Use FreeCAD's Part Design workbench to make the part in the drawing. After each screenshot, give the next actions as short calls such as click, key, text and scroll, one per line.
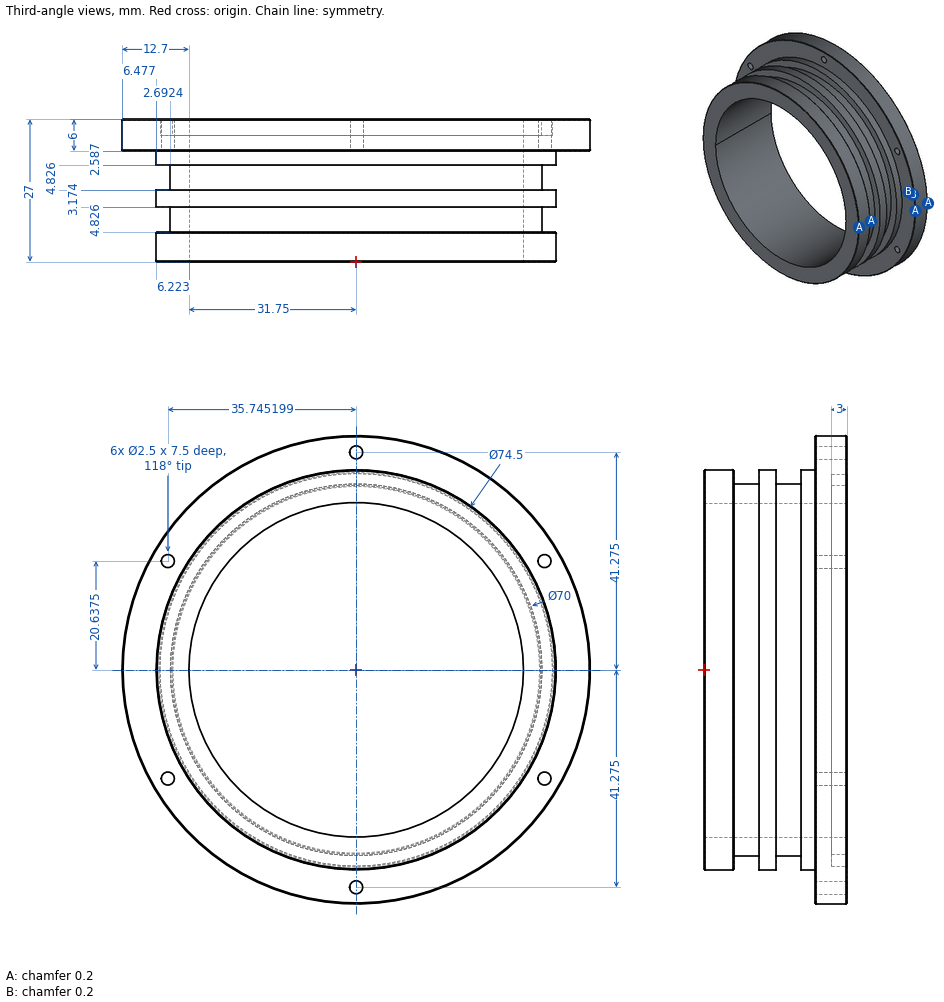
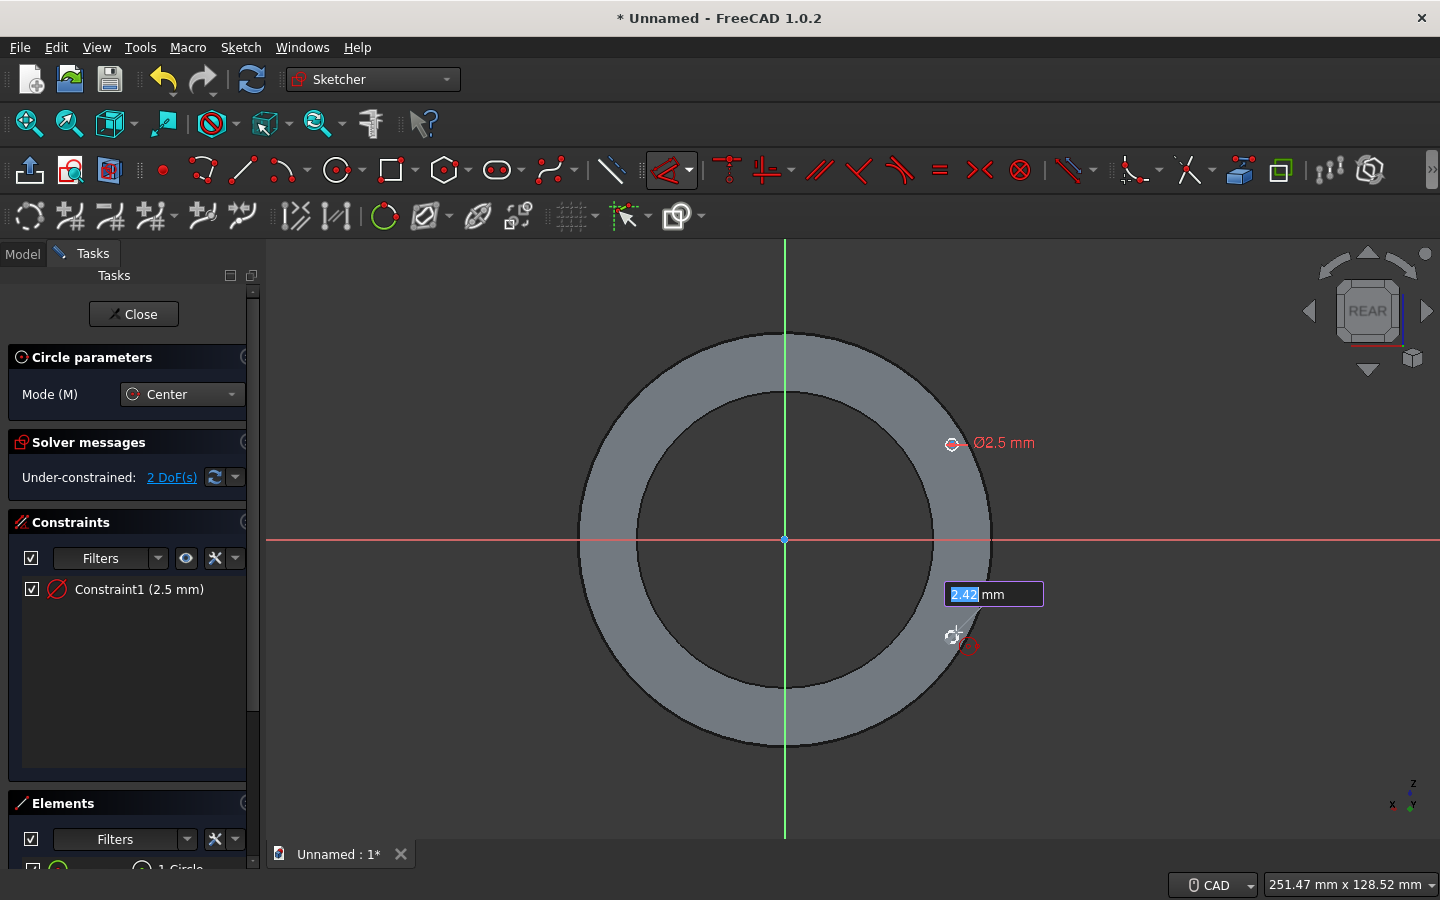
text(2.5)
key(Return)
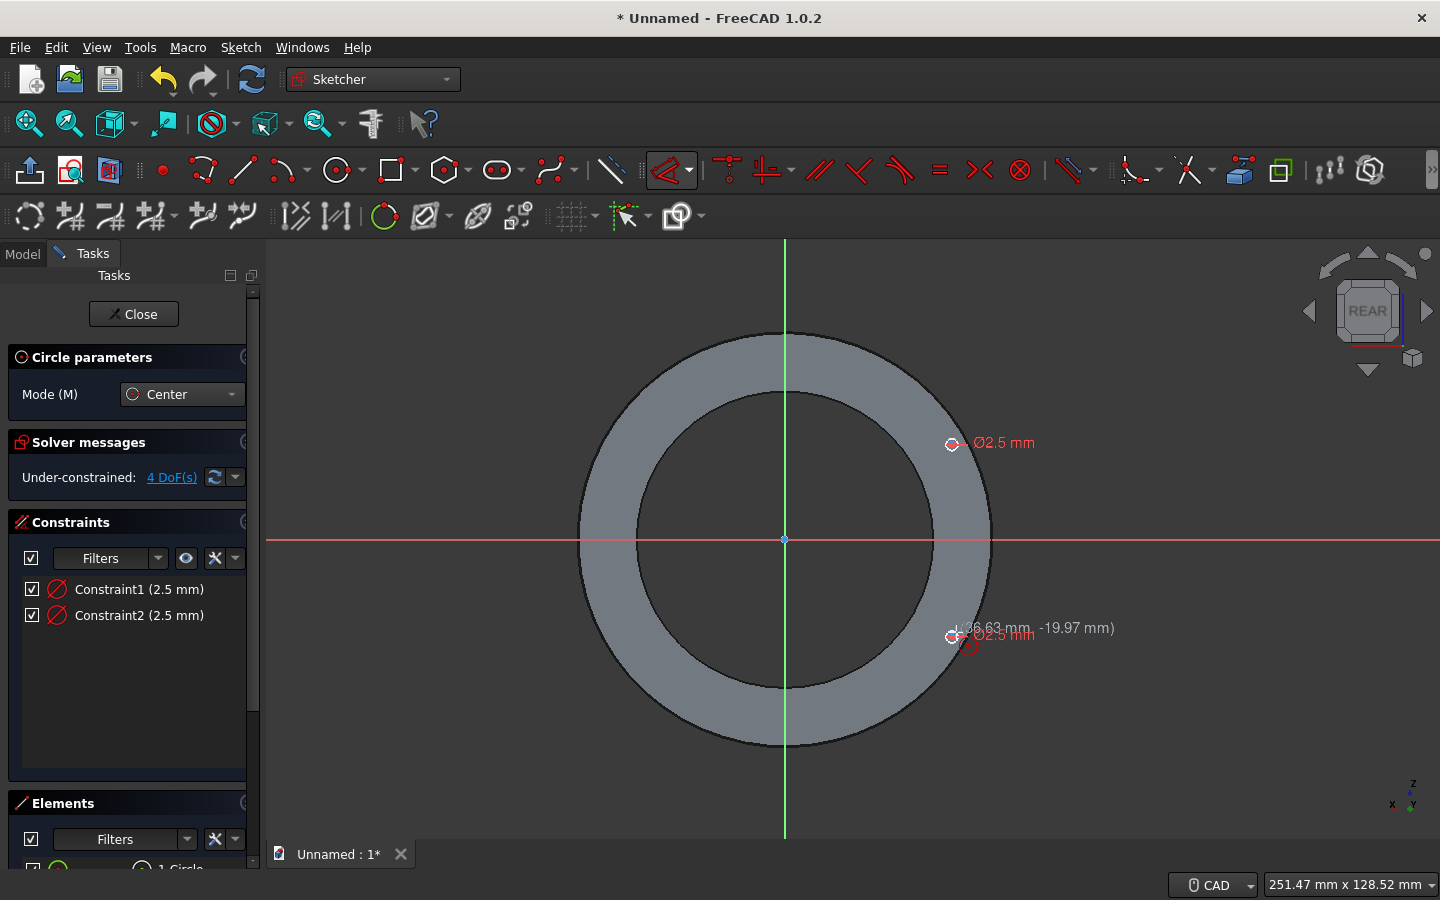
scroll(785, 732, up, 7)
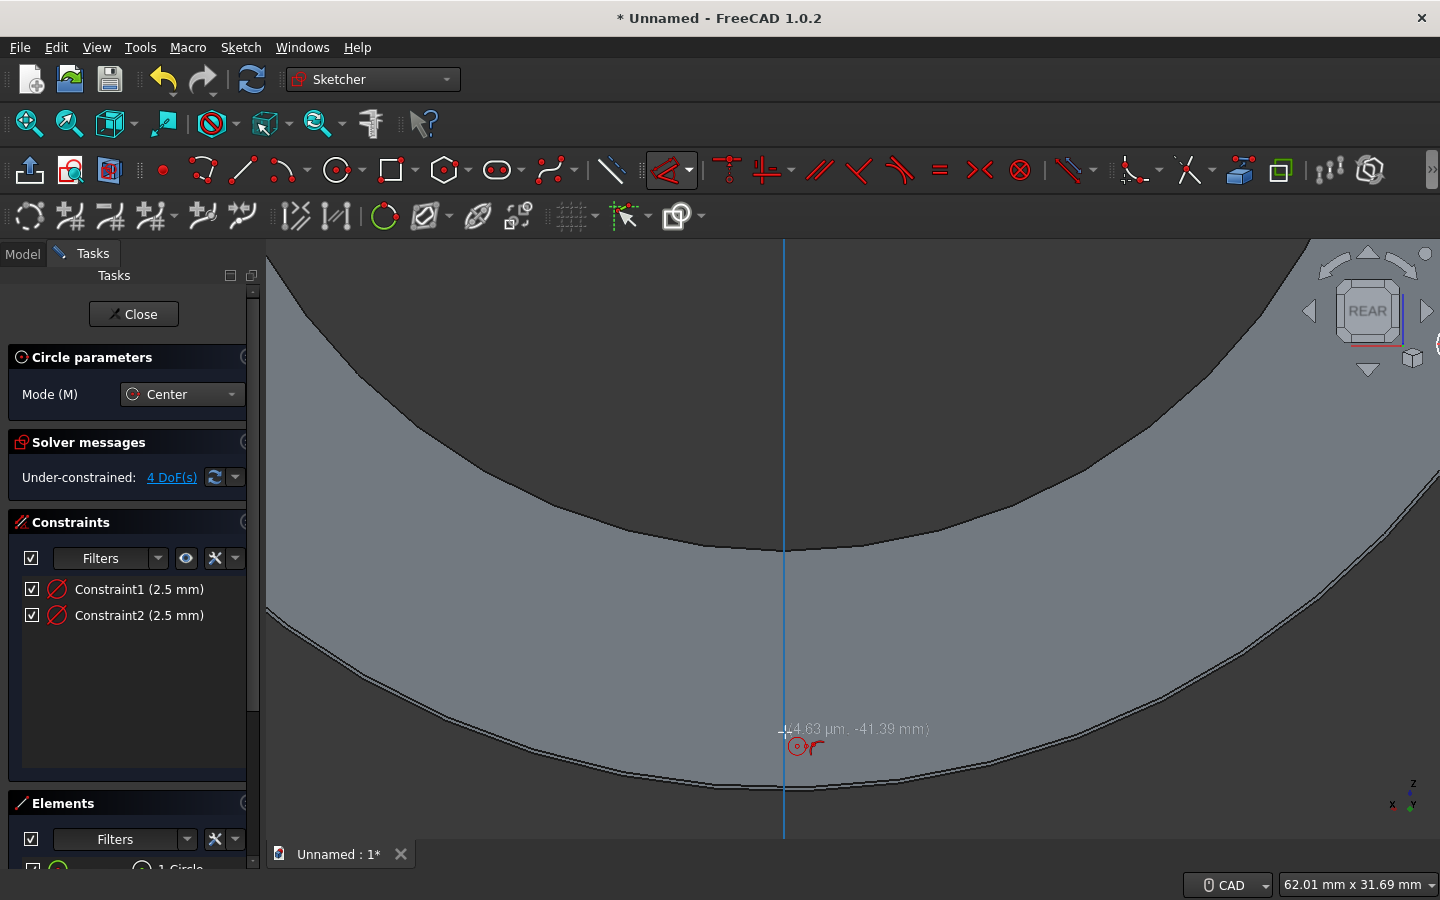
scroll(785, 732, down, 7)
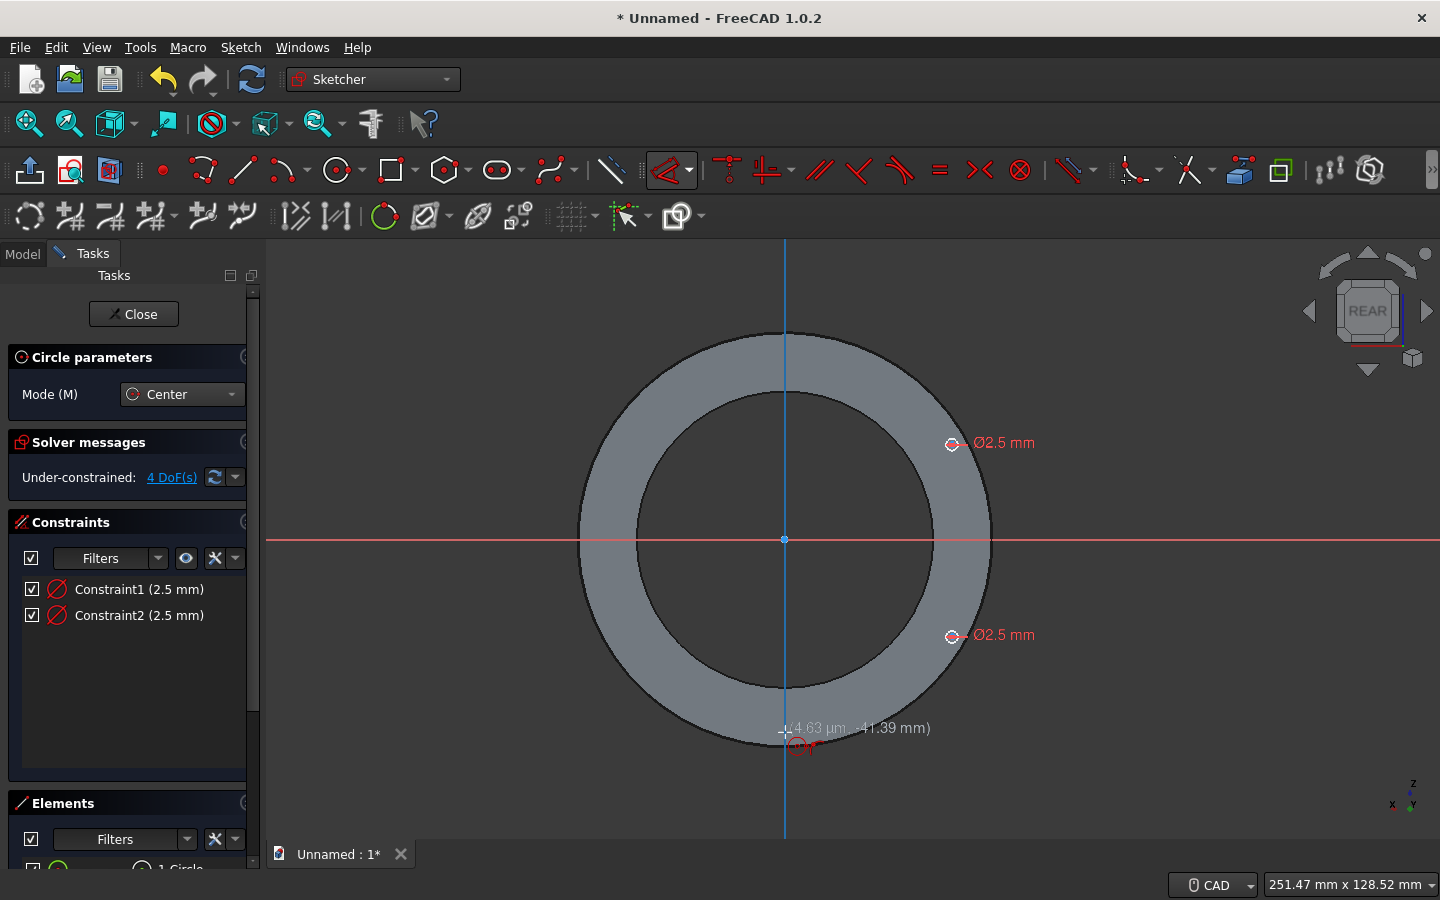
click(785, 732)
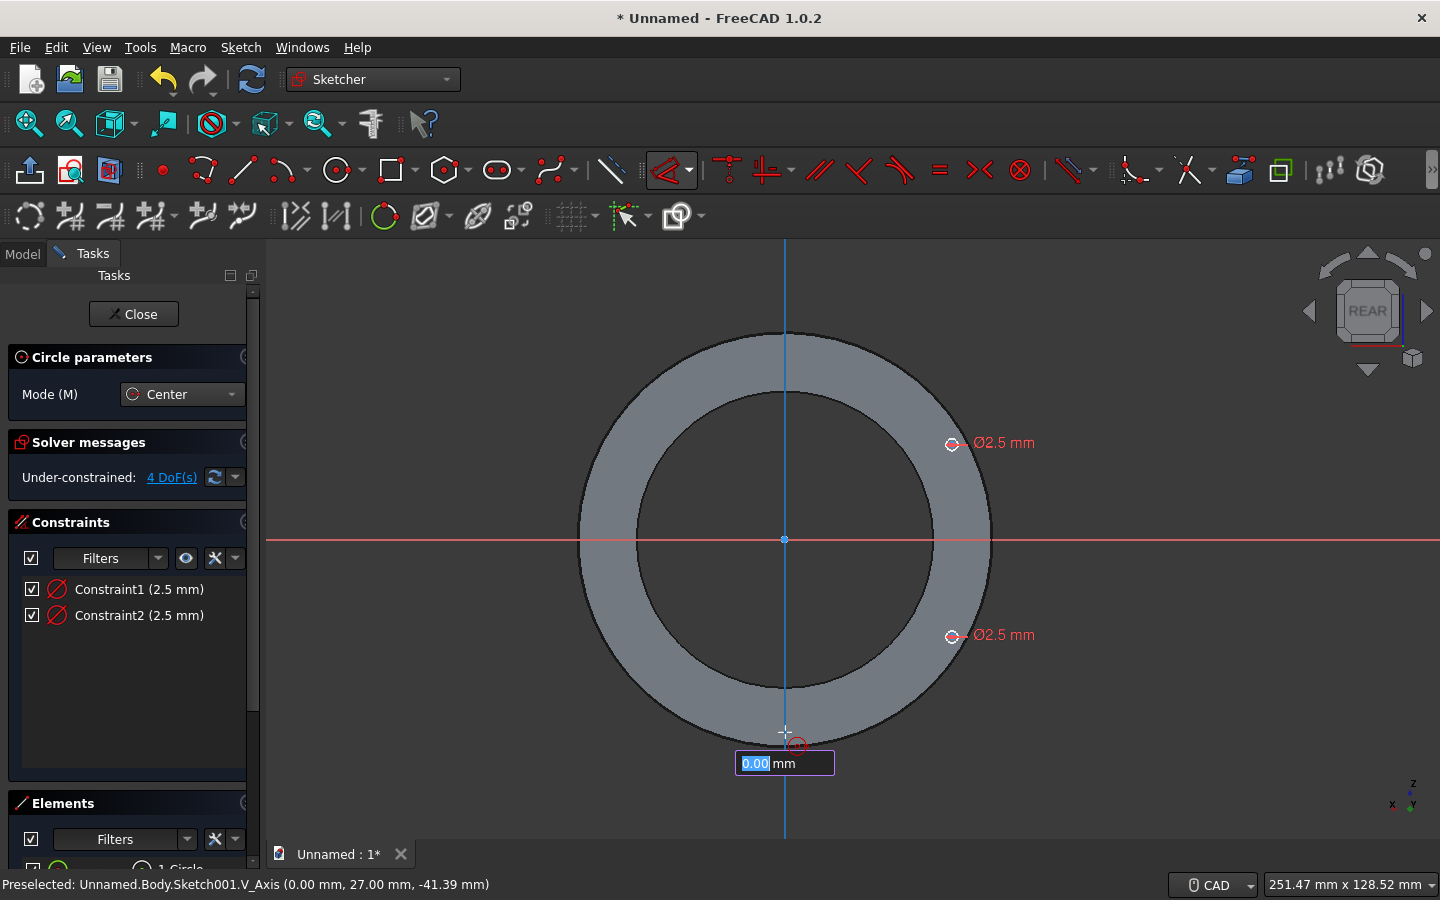
scroll(790, 730, up, 6)
move(790, 730)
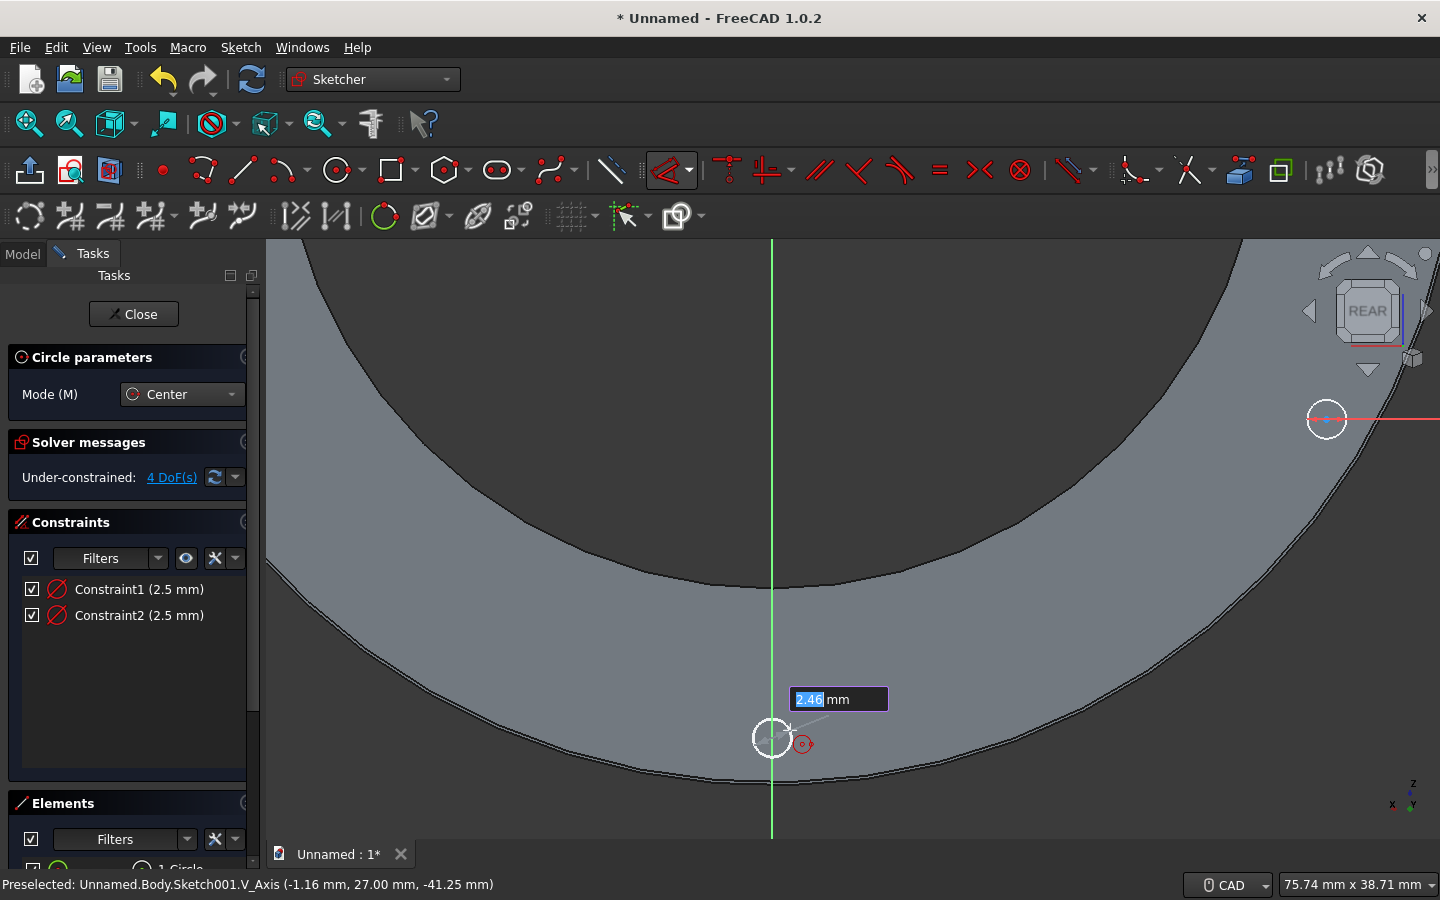
text(2.5)
key(Return)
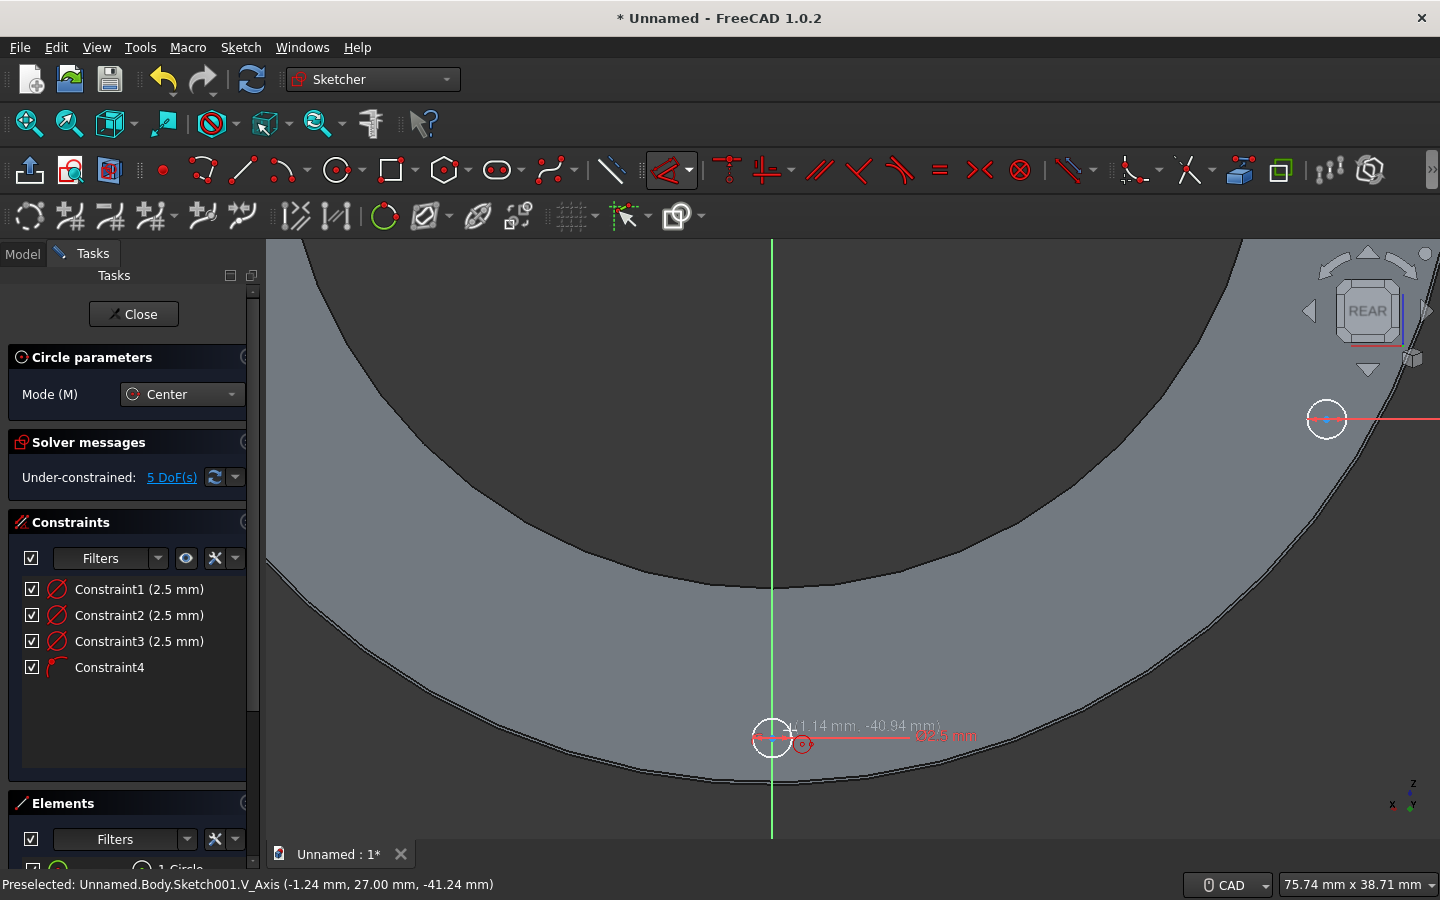
scroll(790, 730, down, 6)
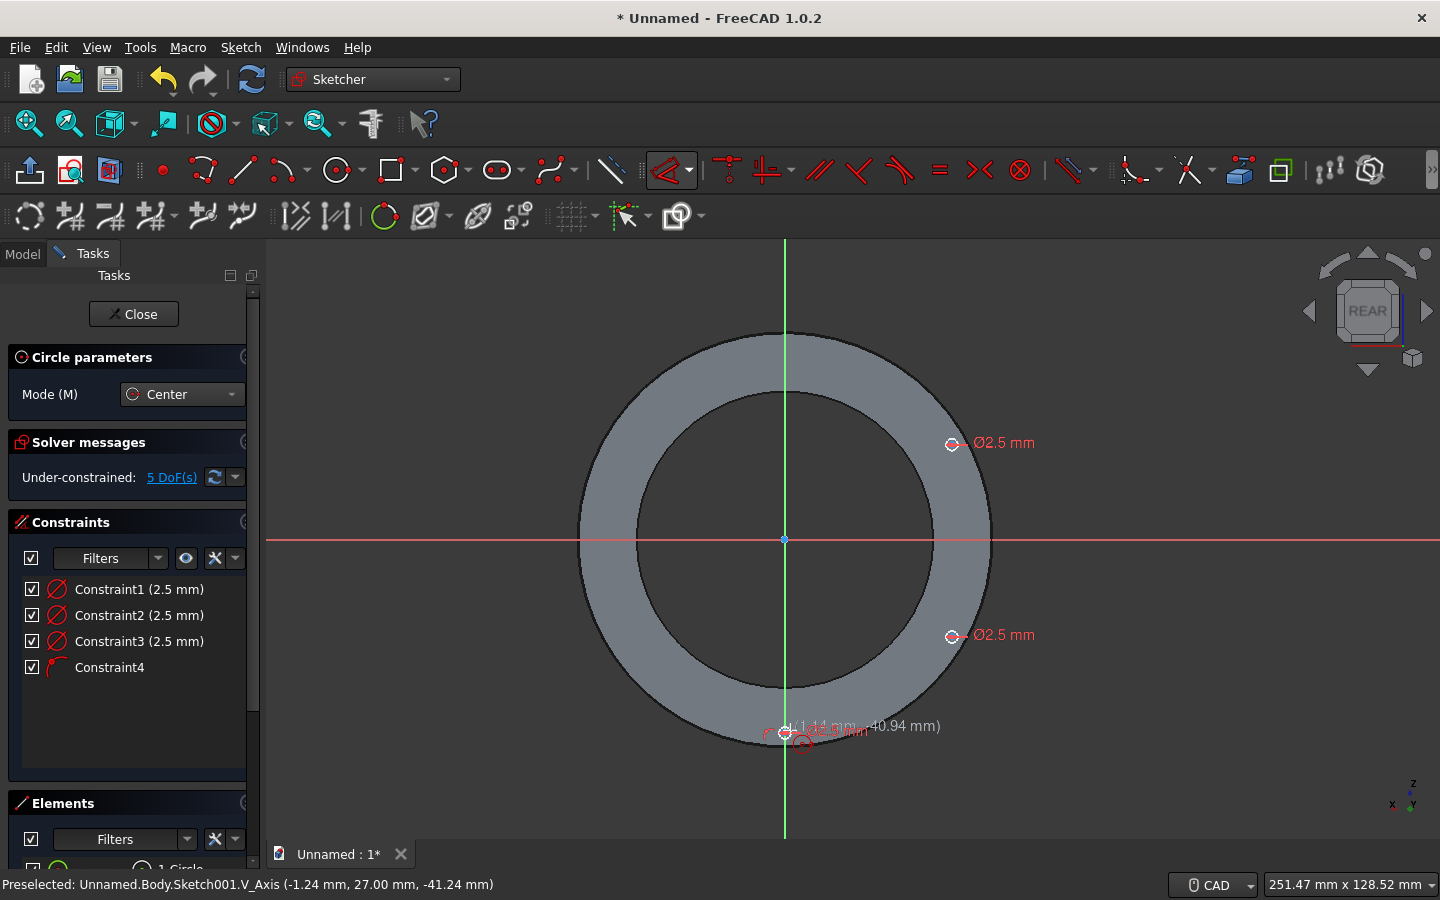
scroll(618, 636, up, 7)